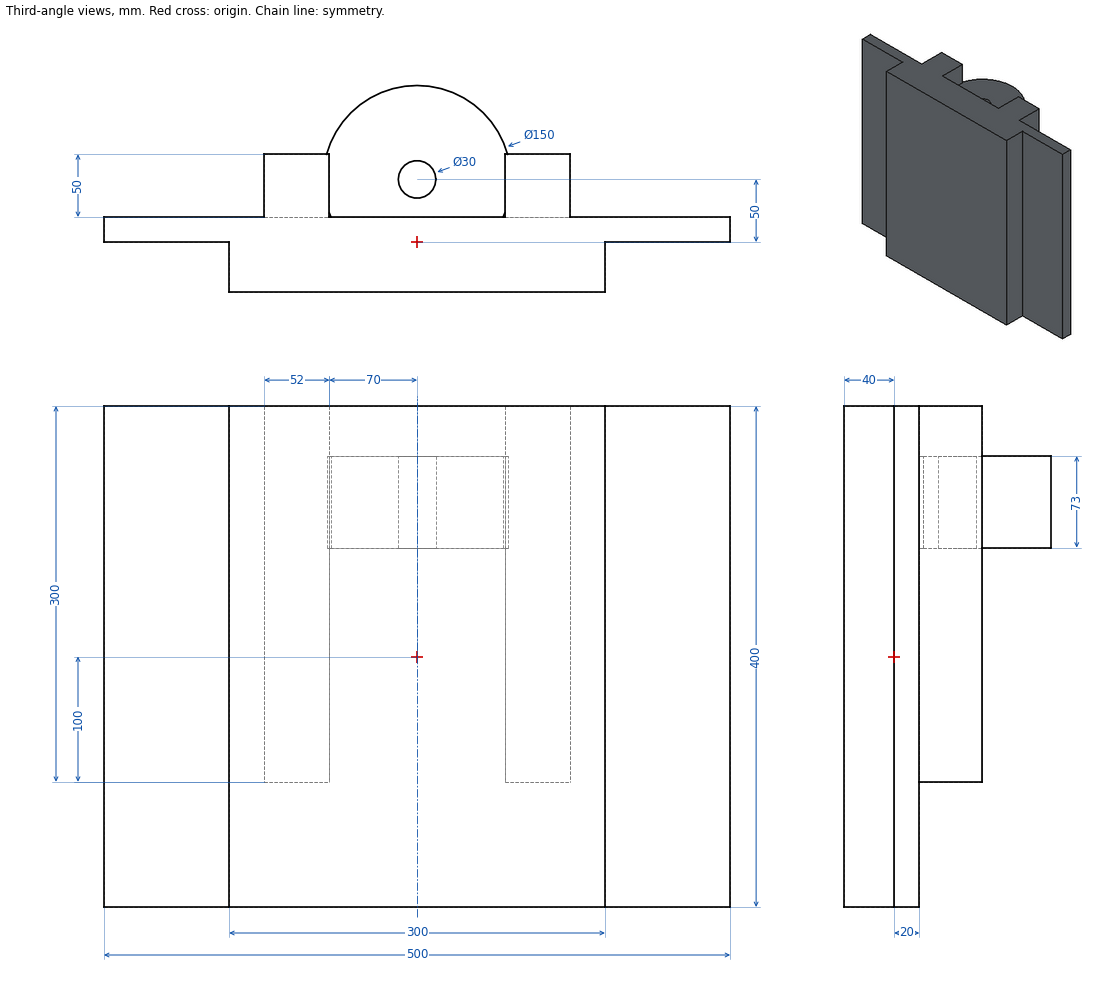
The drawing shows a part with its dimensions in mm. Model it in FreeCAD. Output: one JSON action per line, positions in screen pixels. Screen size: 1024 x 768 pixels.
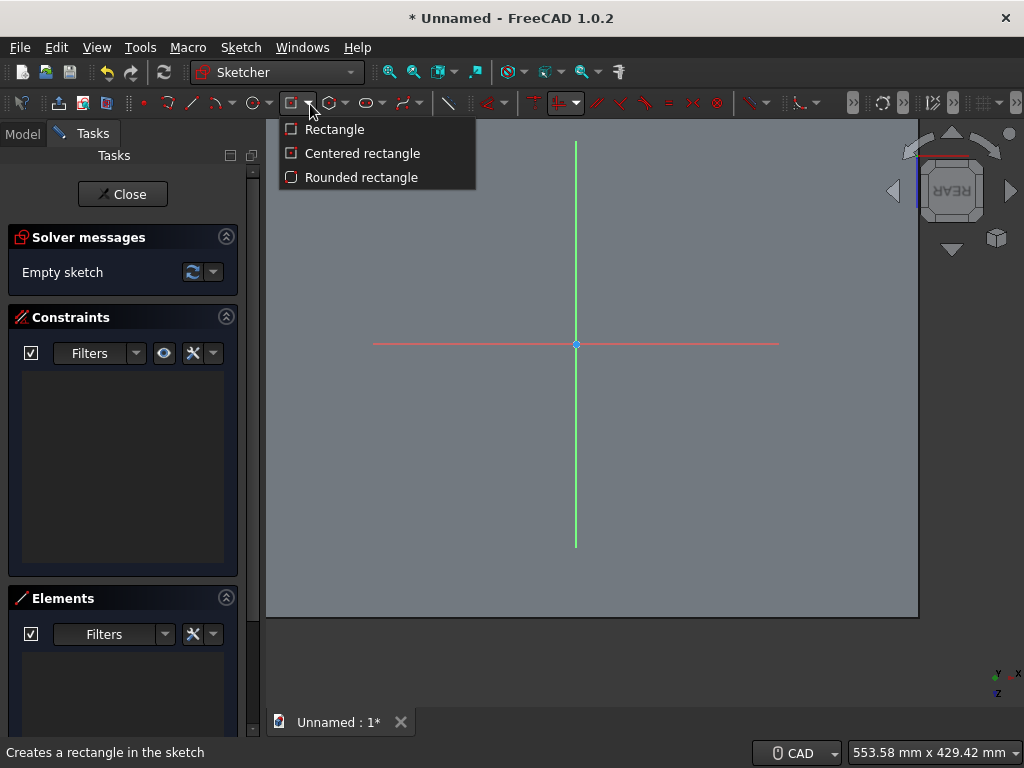
{"action": "left_click", "coordinate": [378, 129]}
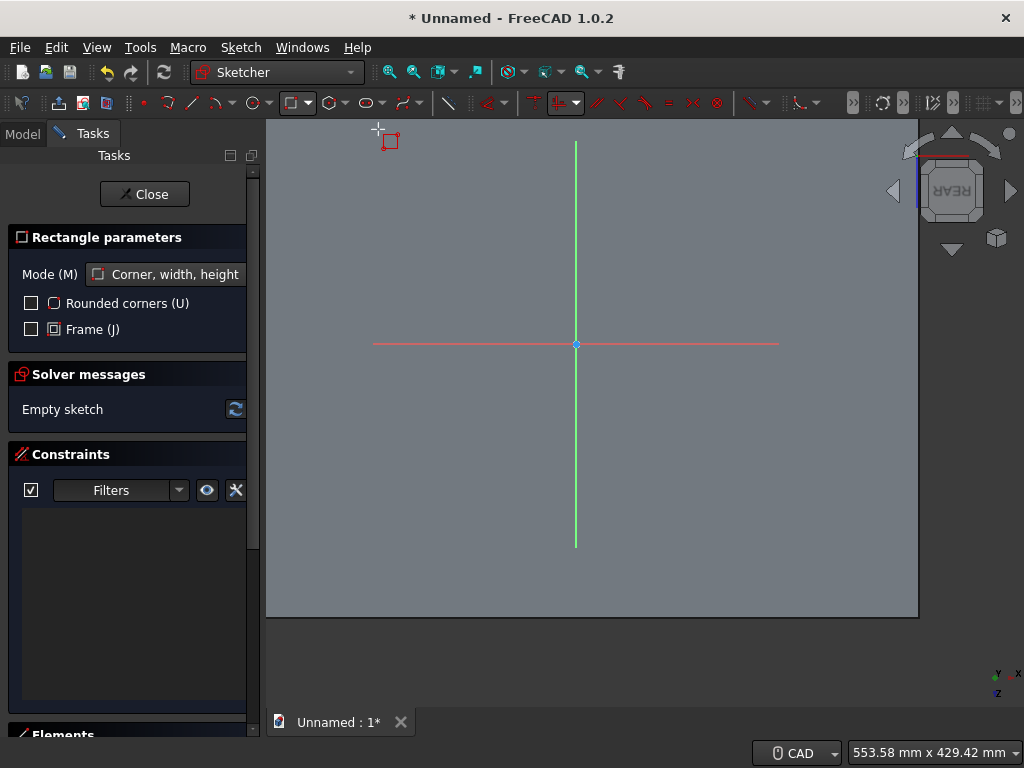
{"action": "left_click", "coordinate": [409, 207]}
{"action": "left_click", "coordinate": [480, 618]}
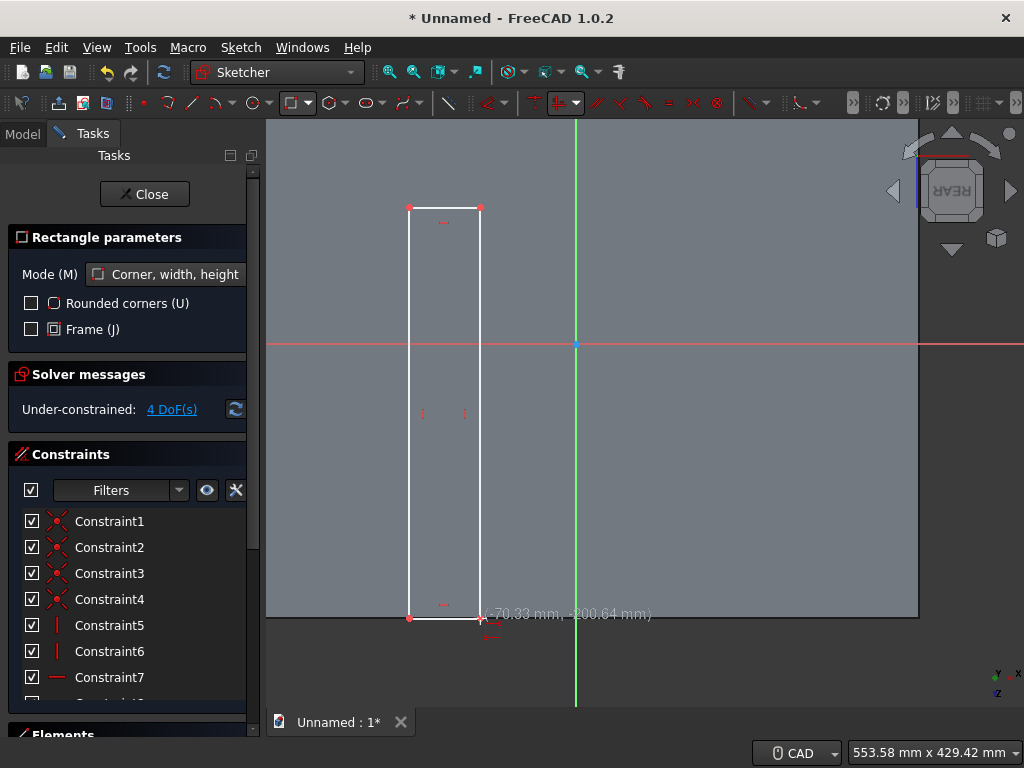
{"action": "left_click", "coordinate": [672, 207]}
{"action": "left_click", "coordinate": [743, 618]}
{"action": "key", "text": "Escape"}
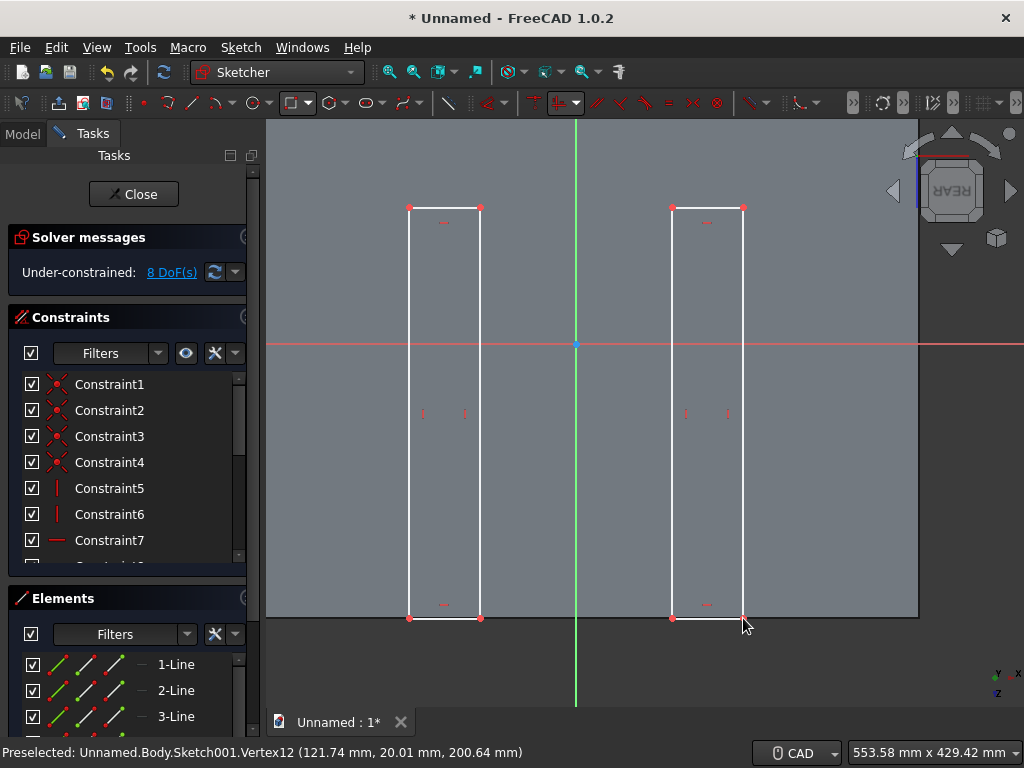
{"action": "left_click", "coordinate": [480, 208]}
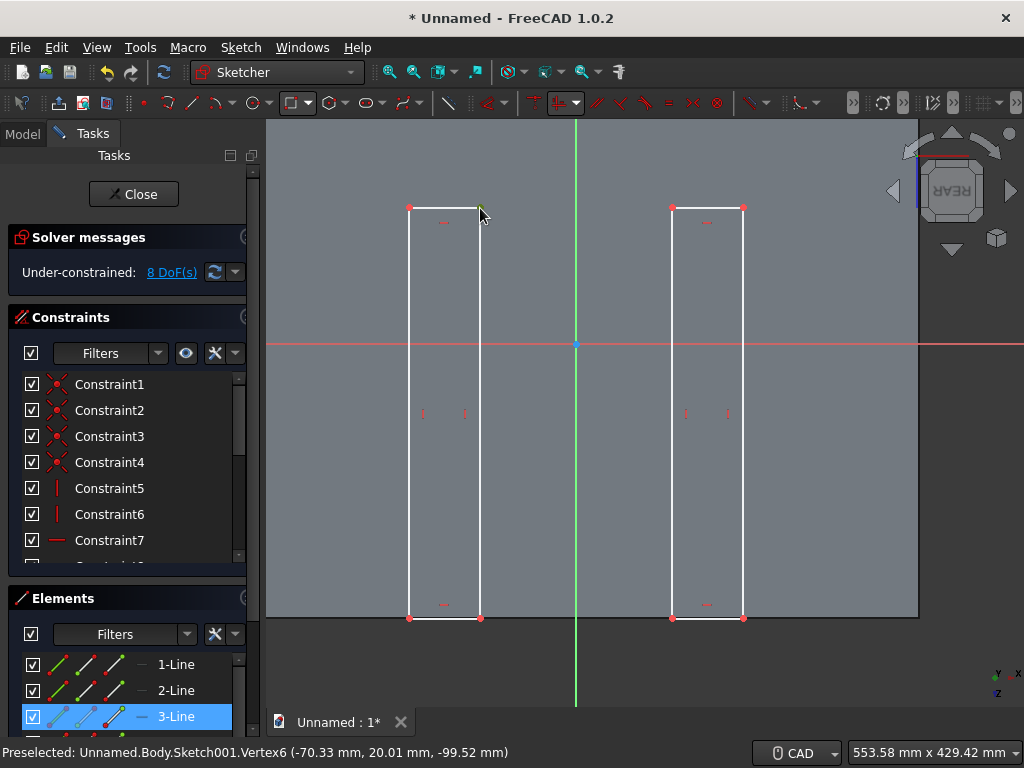
{"action": "left_click", "coordinate": [672, 208]}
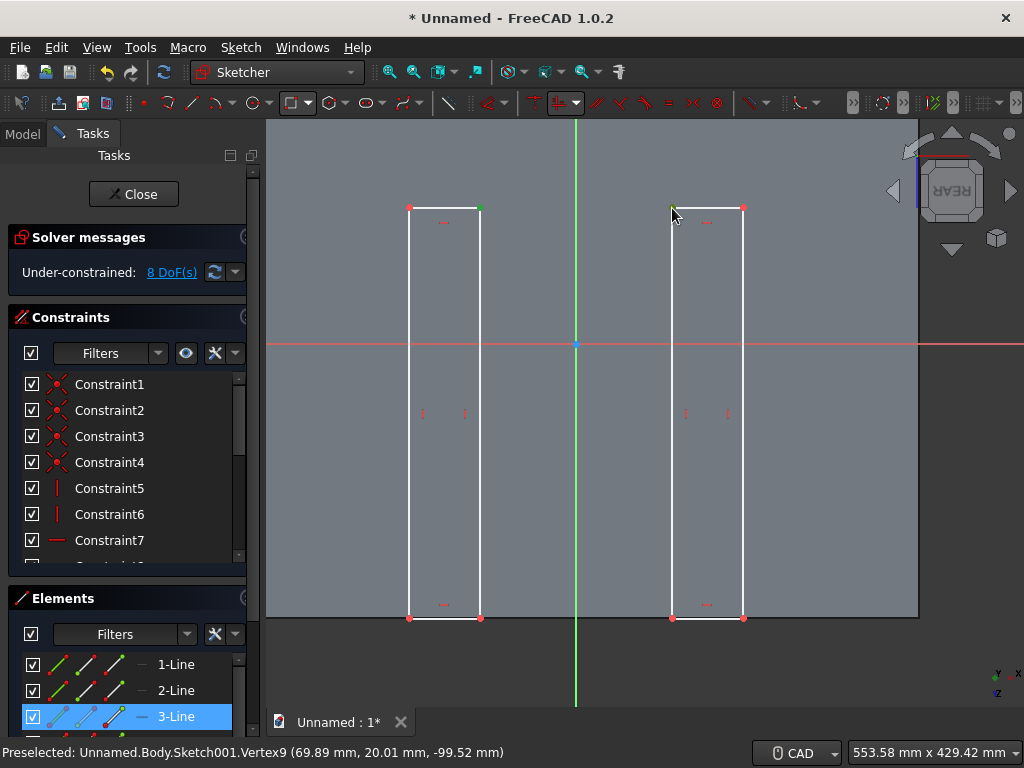
{"action": "left_click", "coordinate": [576, 641]}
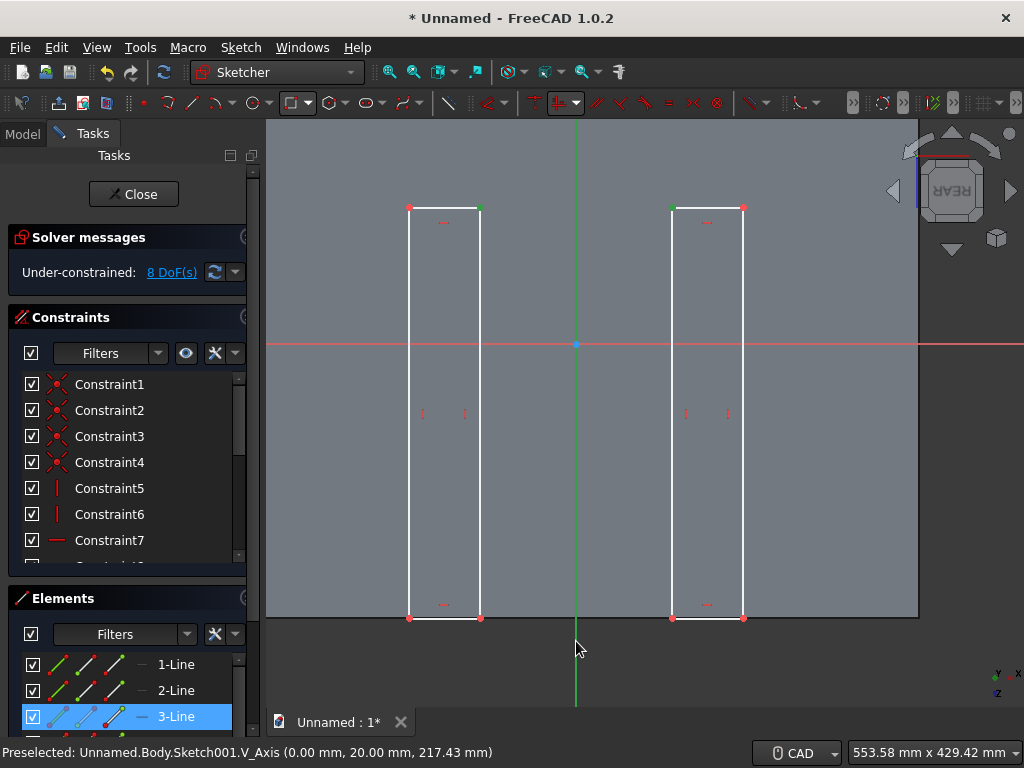
{"action": "left_click", "coordinate": [694, 104]}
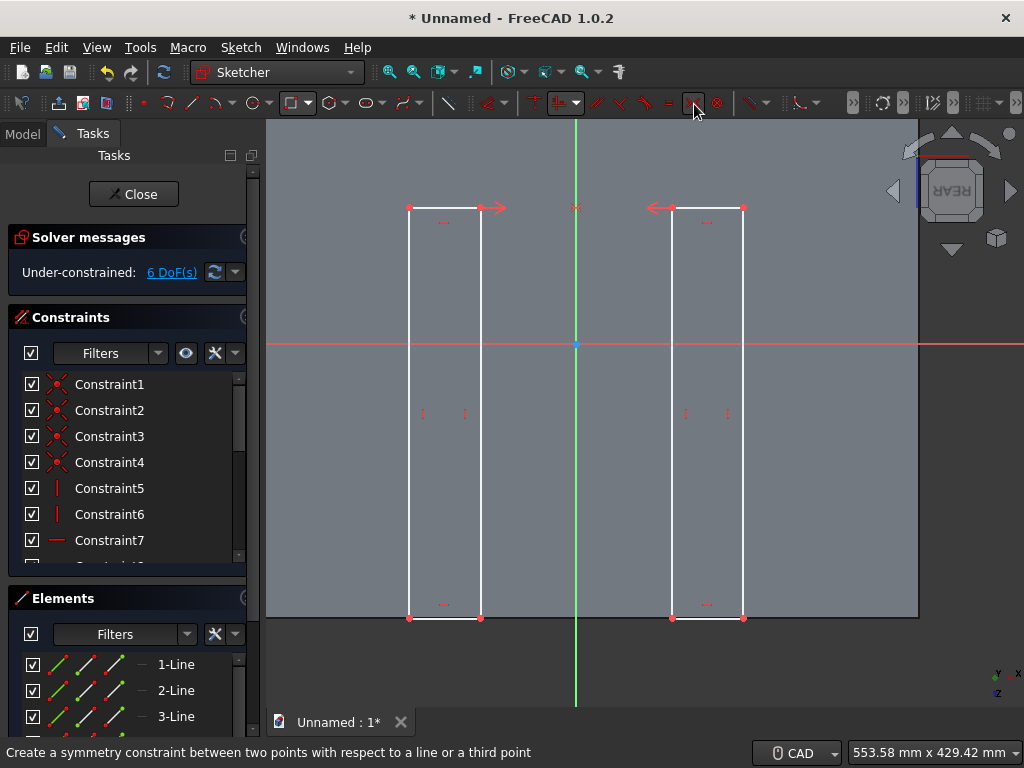
{"action": "left_click", "coordinate": [409, 619]}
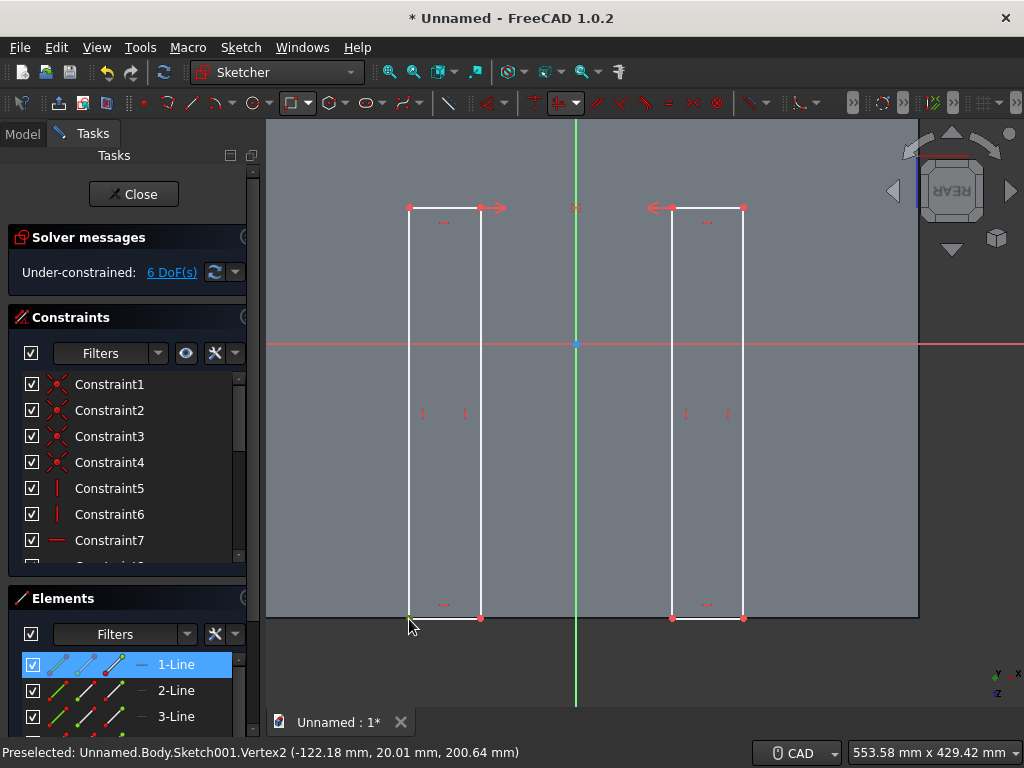
{"action": "left_click", "coordinate": [743, 619]}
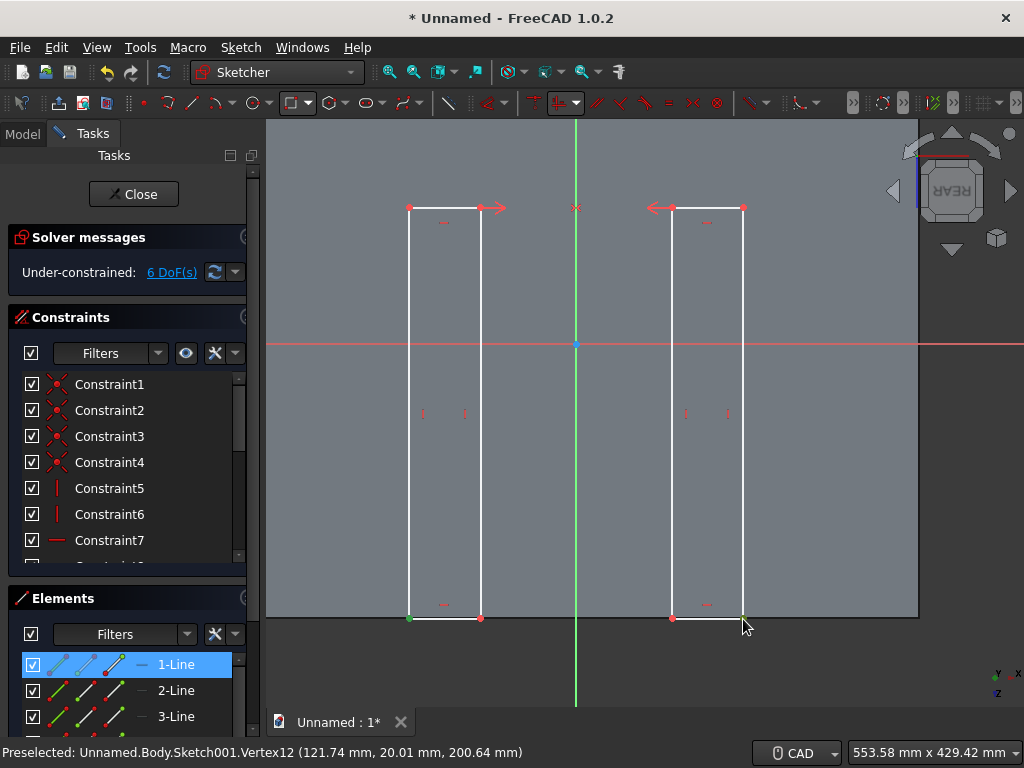
{"action": "left_click", "coordinate": [576, 641]}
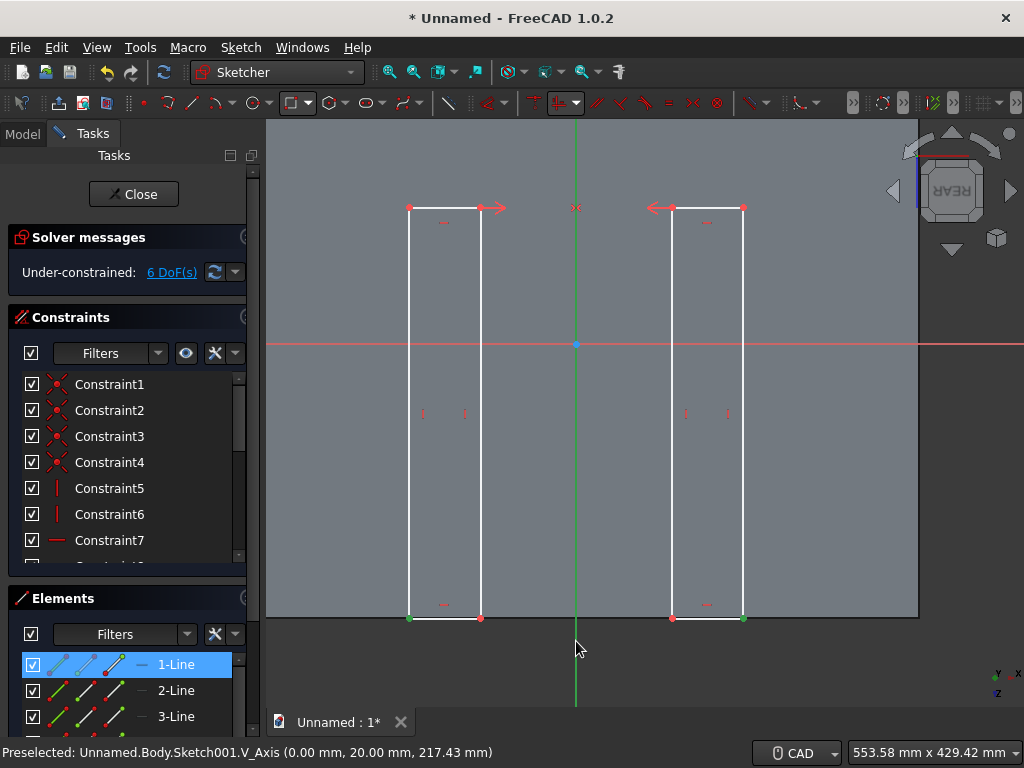
{"action": "left_click", "coordinate": [694, 104]}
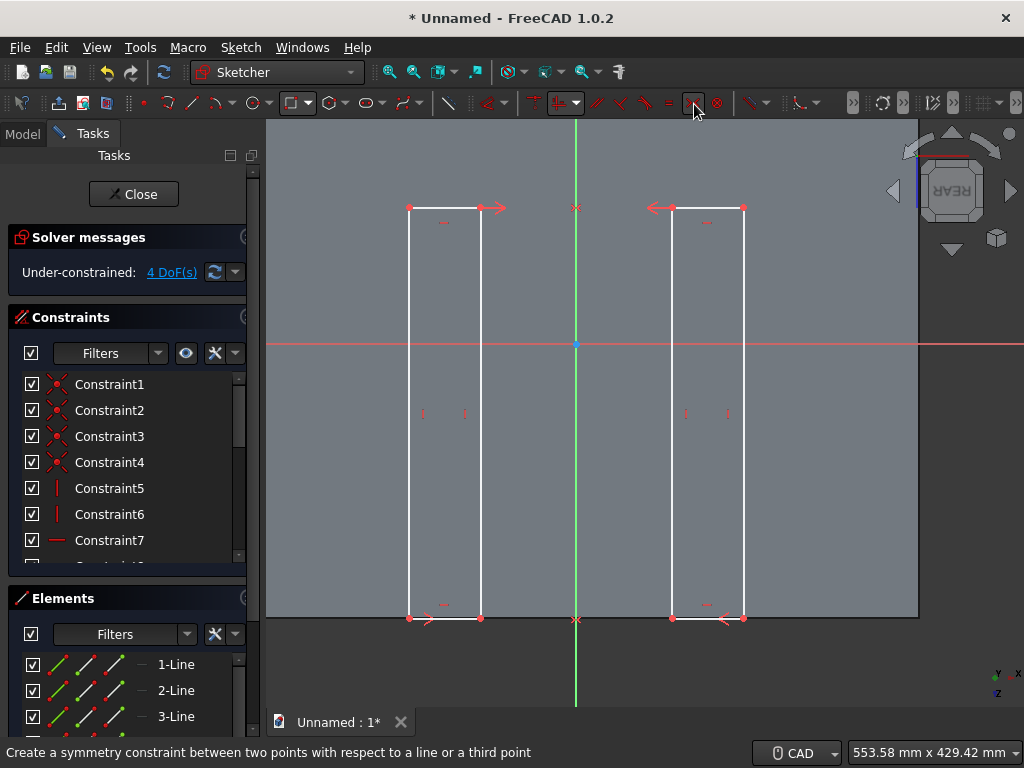
{"action": "left_click", "coordinate": [488, 104]}